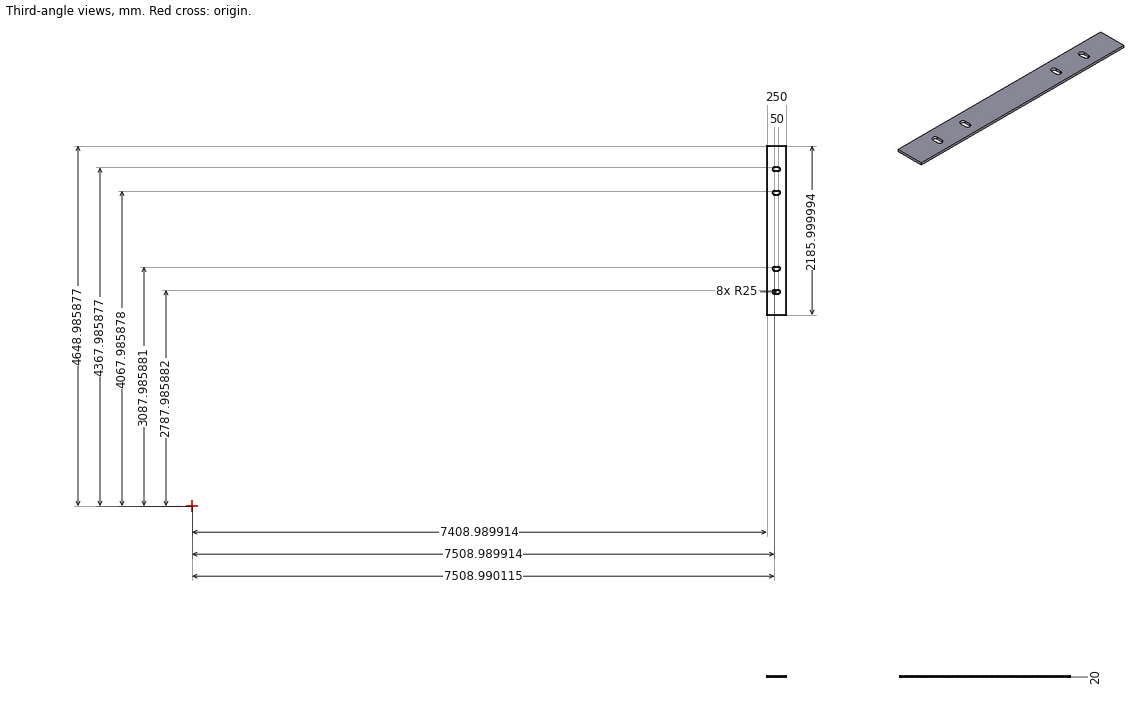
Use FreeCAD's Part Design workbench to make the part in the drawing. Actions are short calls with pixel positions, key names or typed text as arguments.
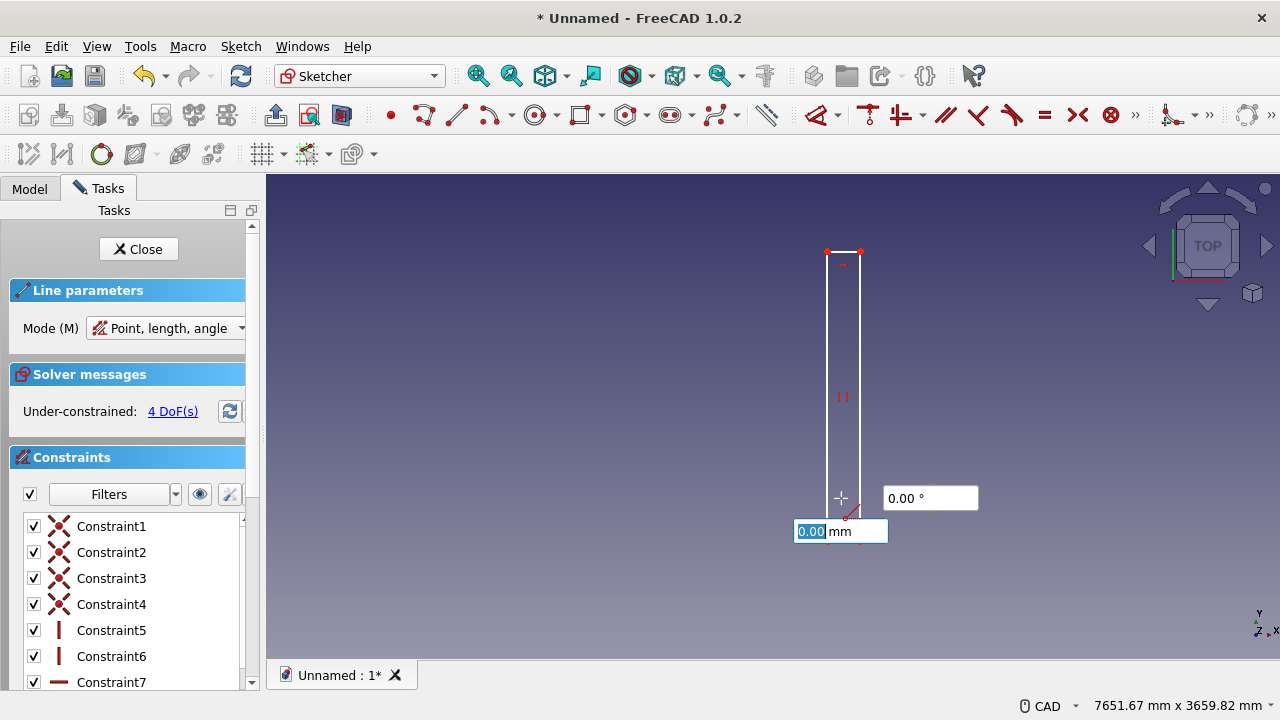
scroll(847, 498, up, 5)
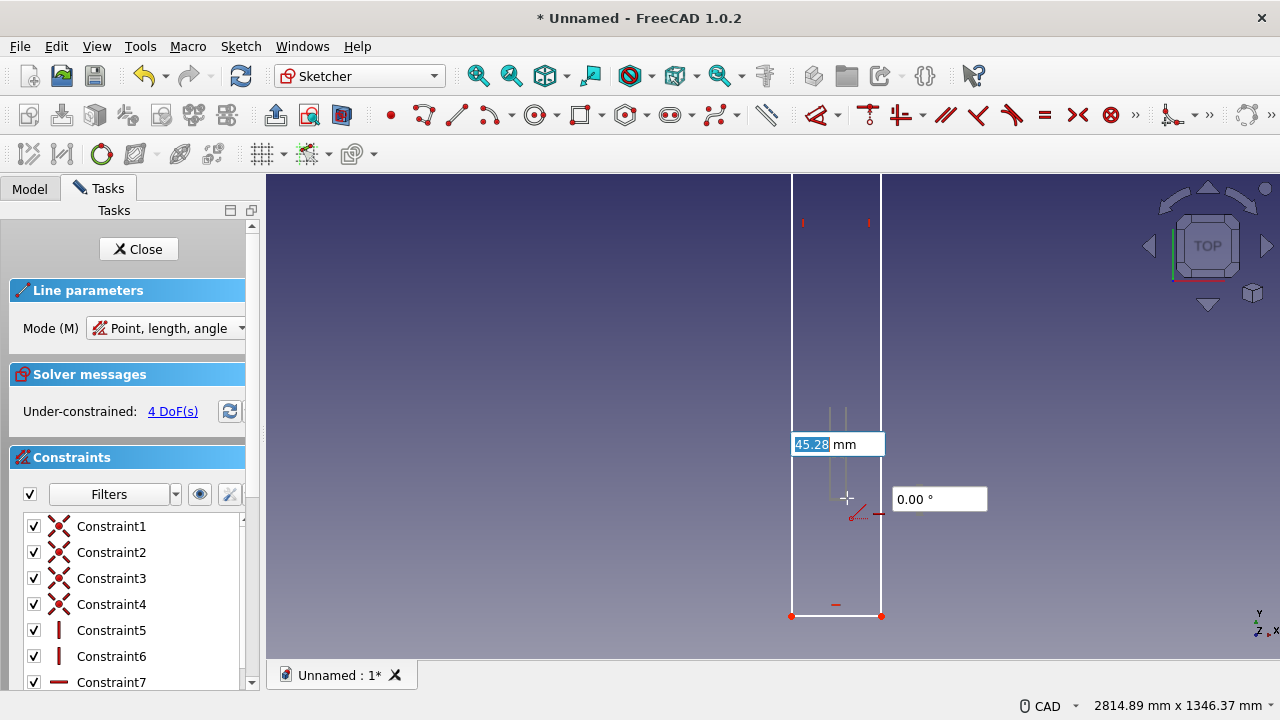
click(847, 497)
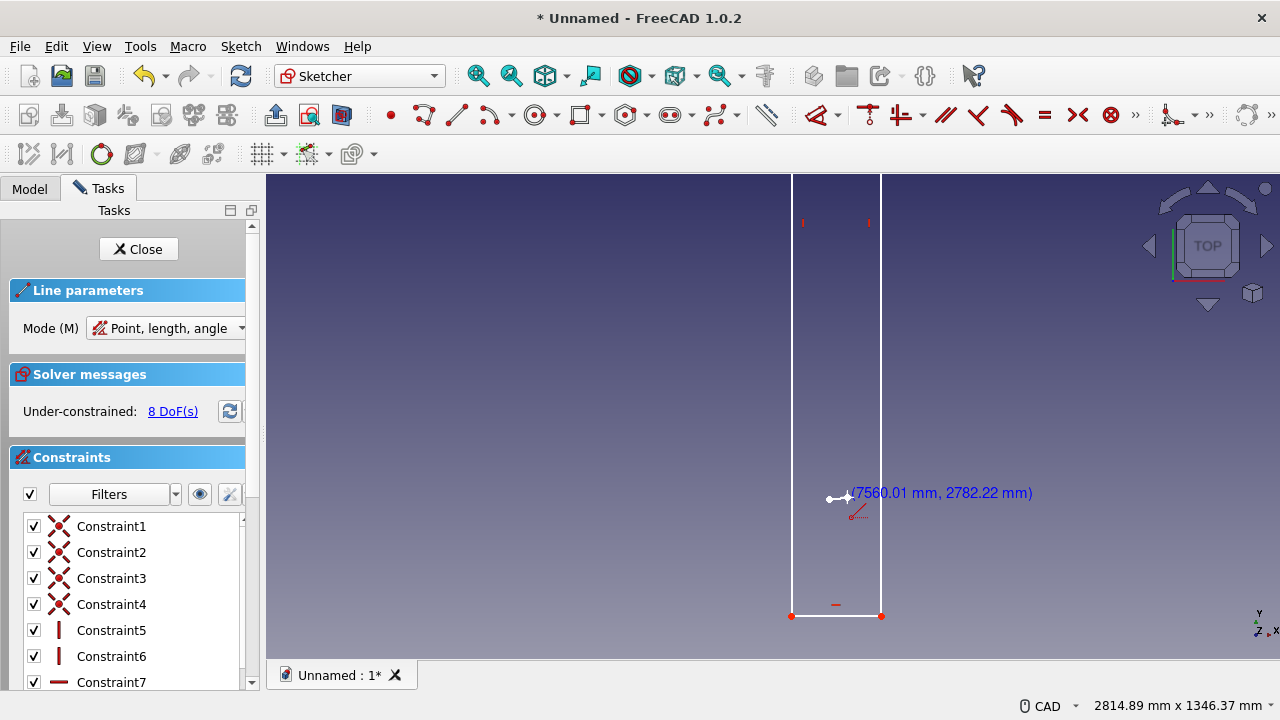
click(847, 514)
click(829, 514)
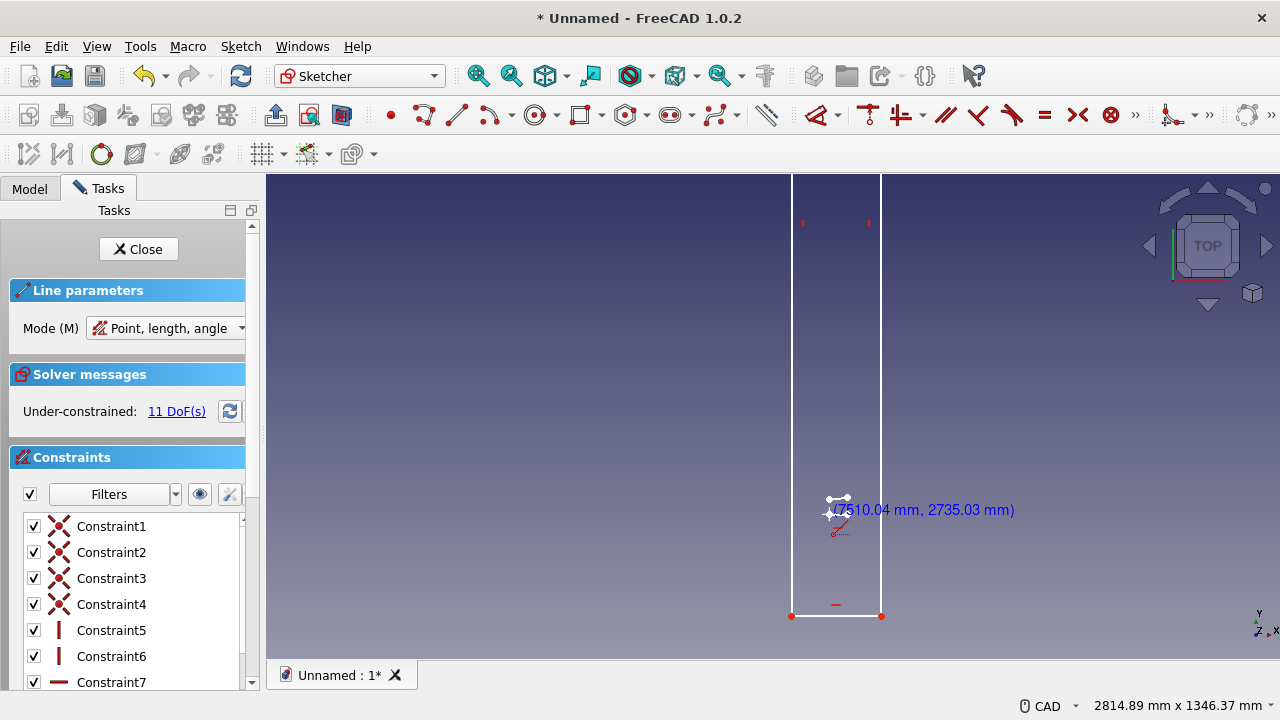
click(512, 116)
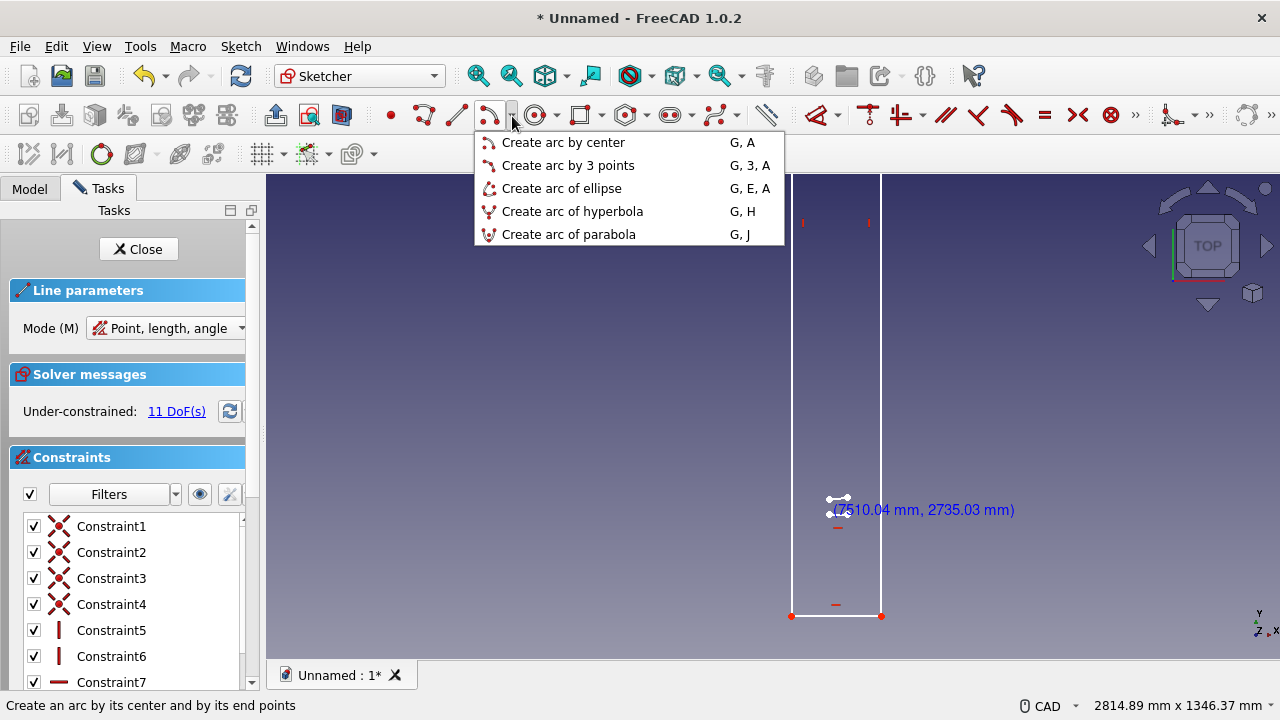
click(630, 166)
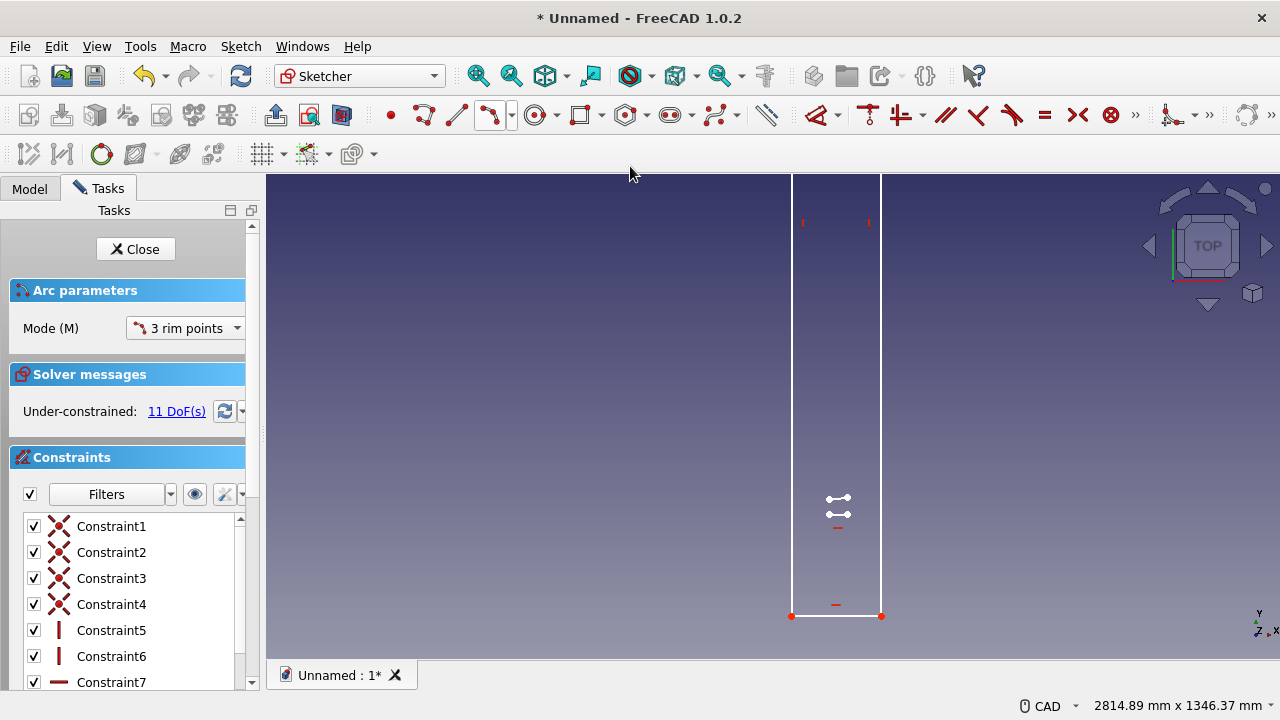
scroll(847, 496, up, 3)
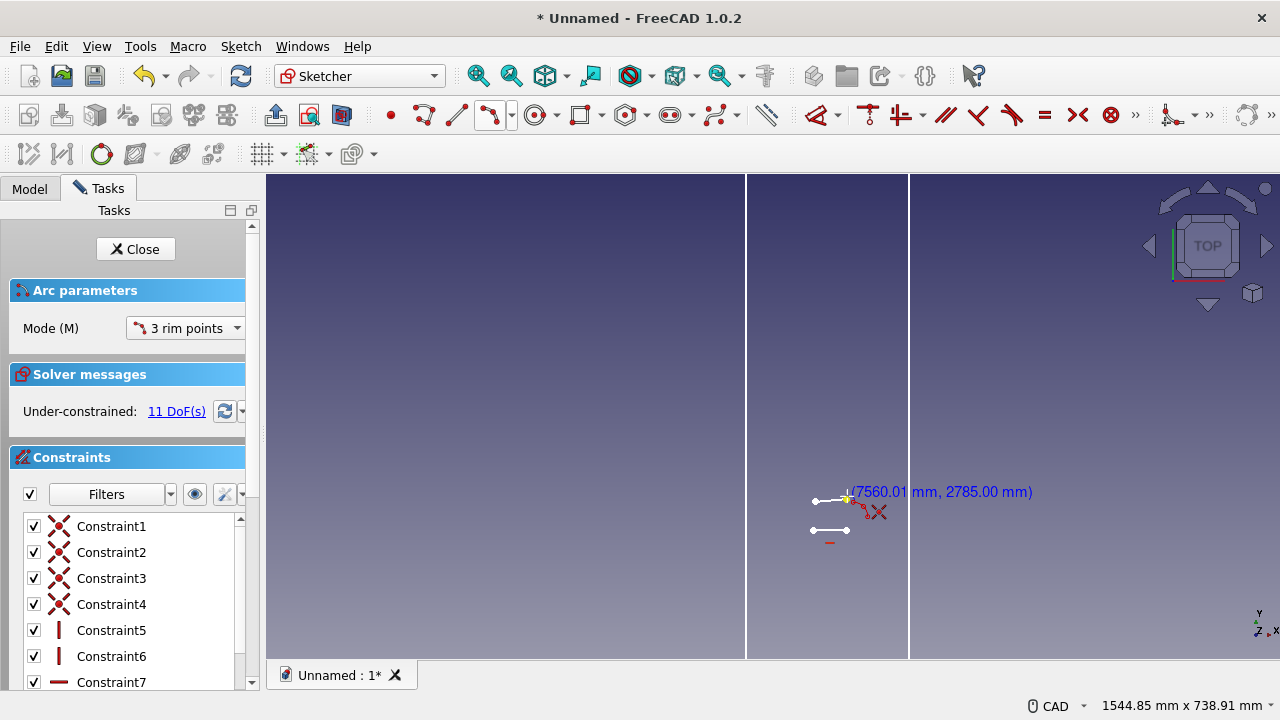
click(847, 499)
click(847, 530)
click(862, 512)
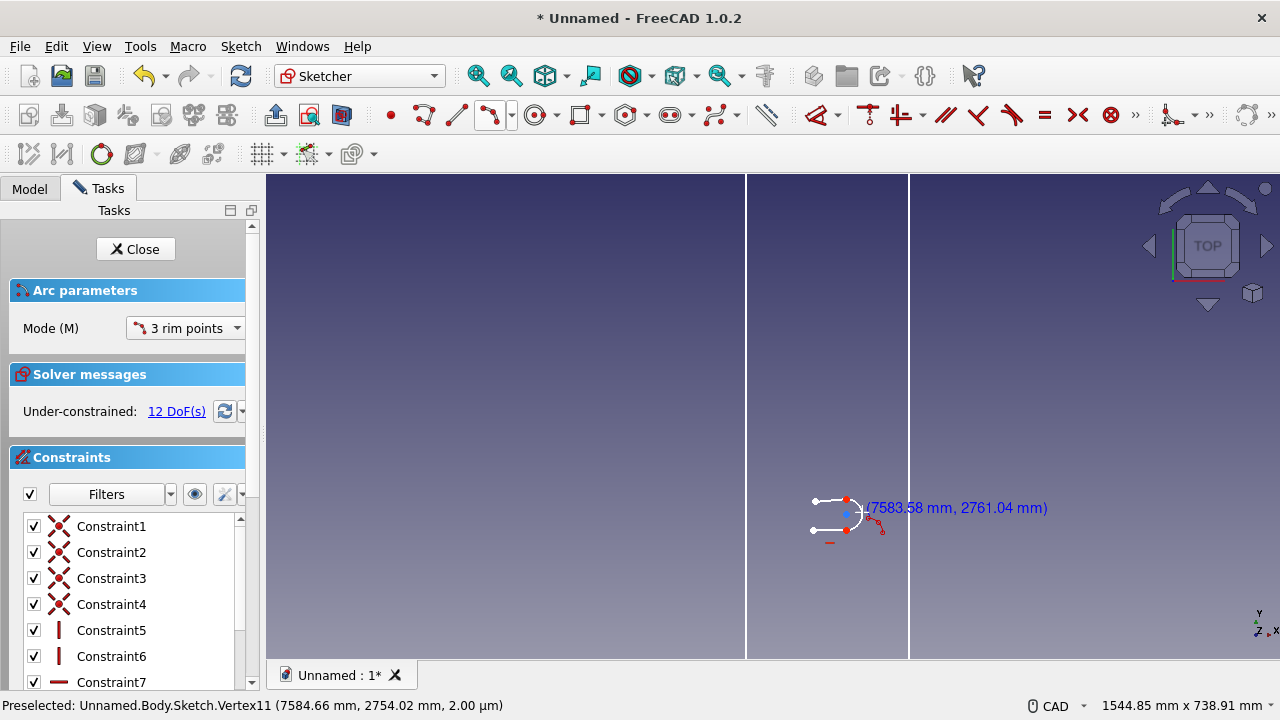
click(814, 530)
click(815, 502)
click(797, 512)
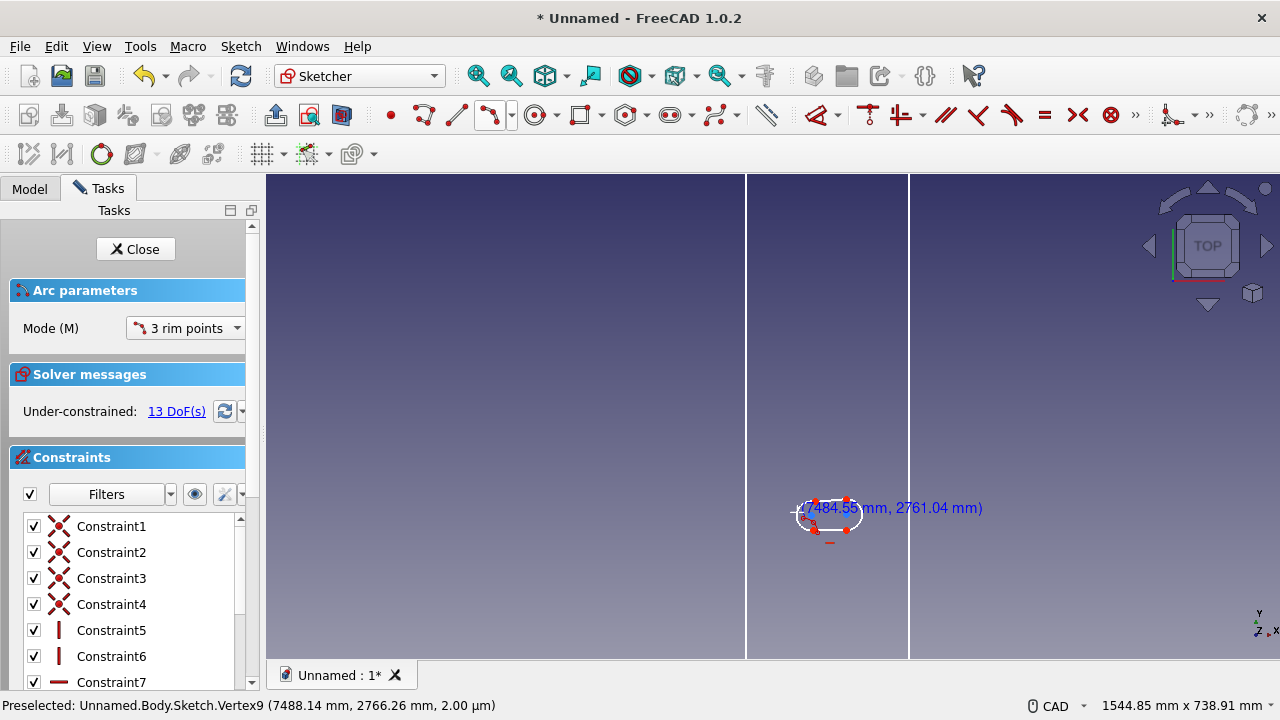
key(g)
key(l)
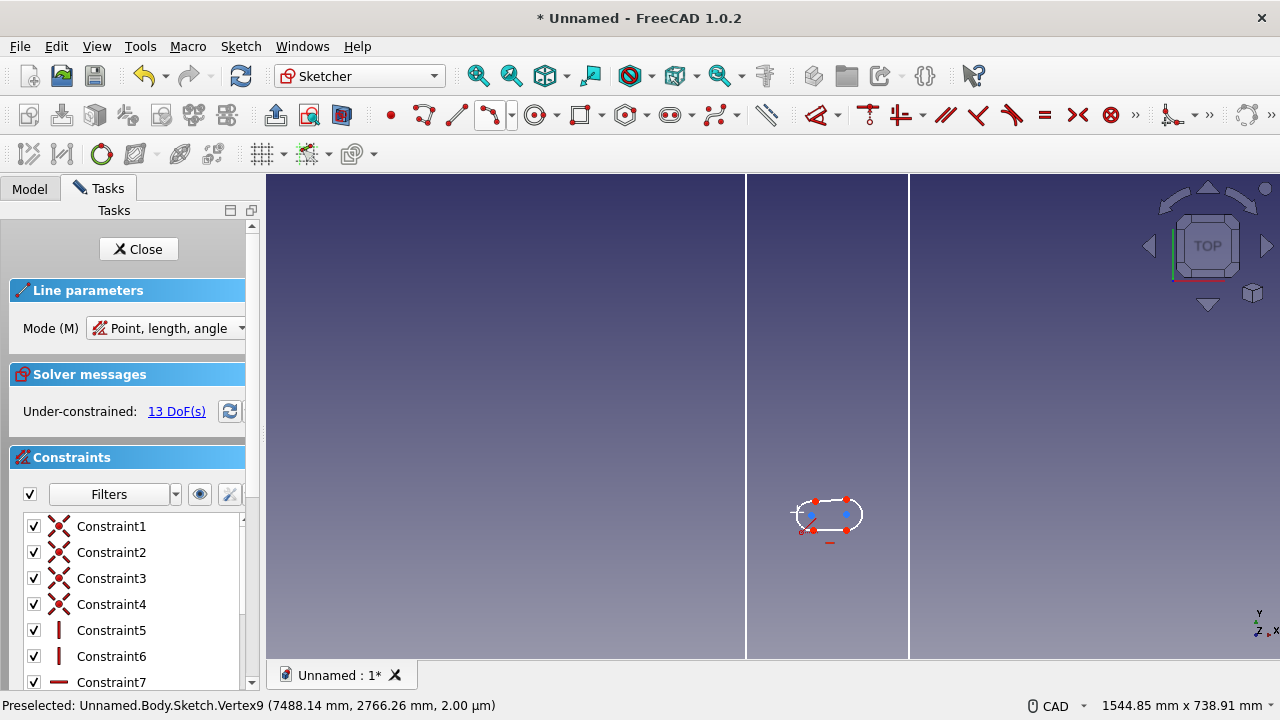
scroll(673, 524, down, 8)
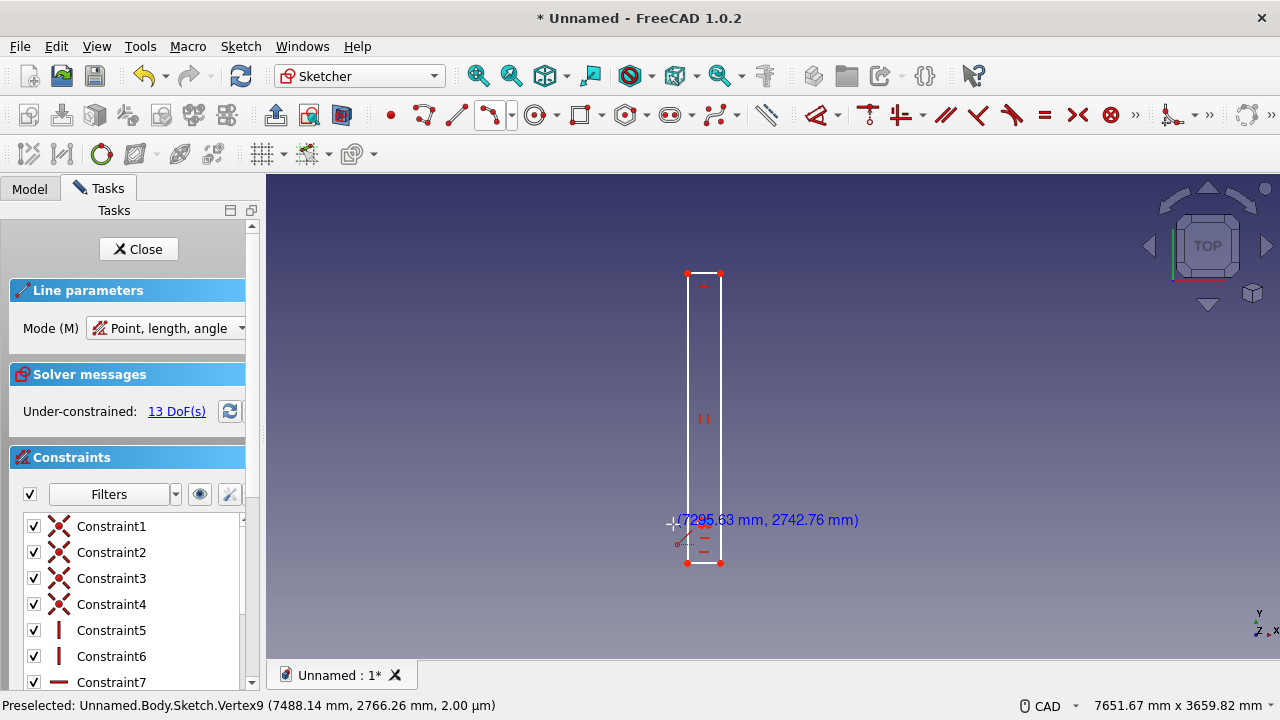
click(702, 479)